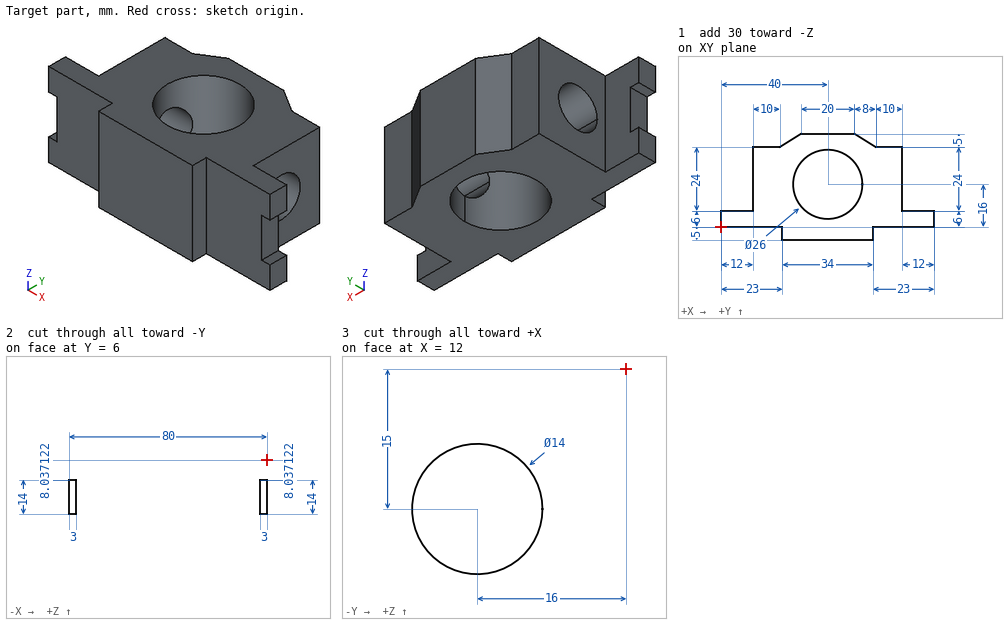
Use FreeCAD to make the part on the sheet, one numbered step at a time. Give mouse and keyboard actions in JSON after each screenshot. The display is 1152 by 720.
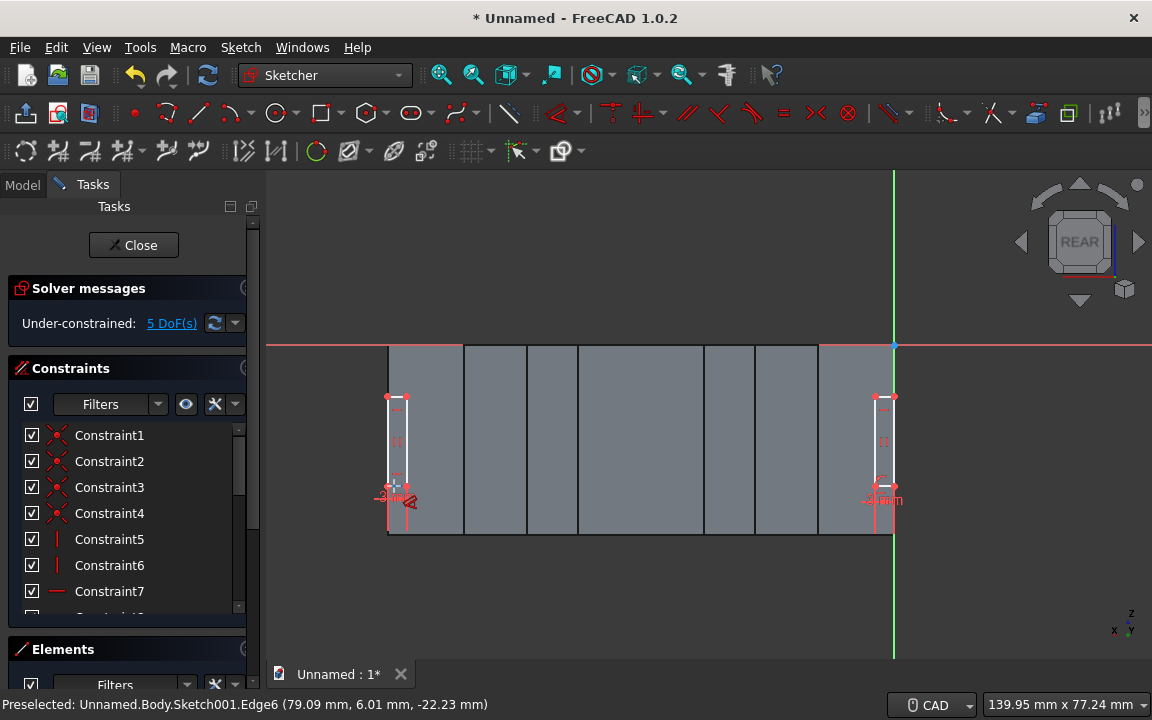
{"action": "left_click", "coordinate": [875, 424]}
{"action": "left_click", "coordinate": [909, 442]}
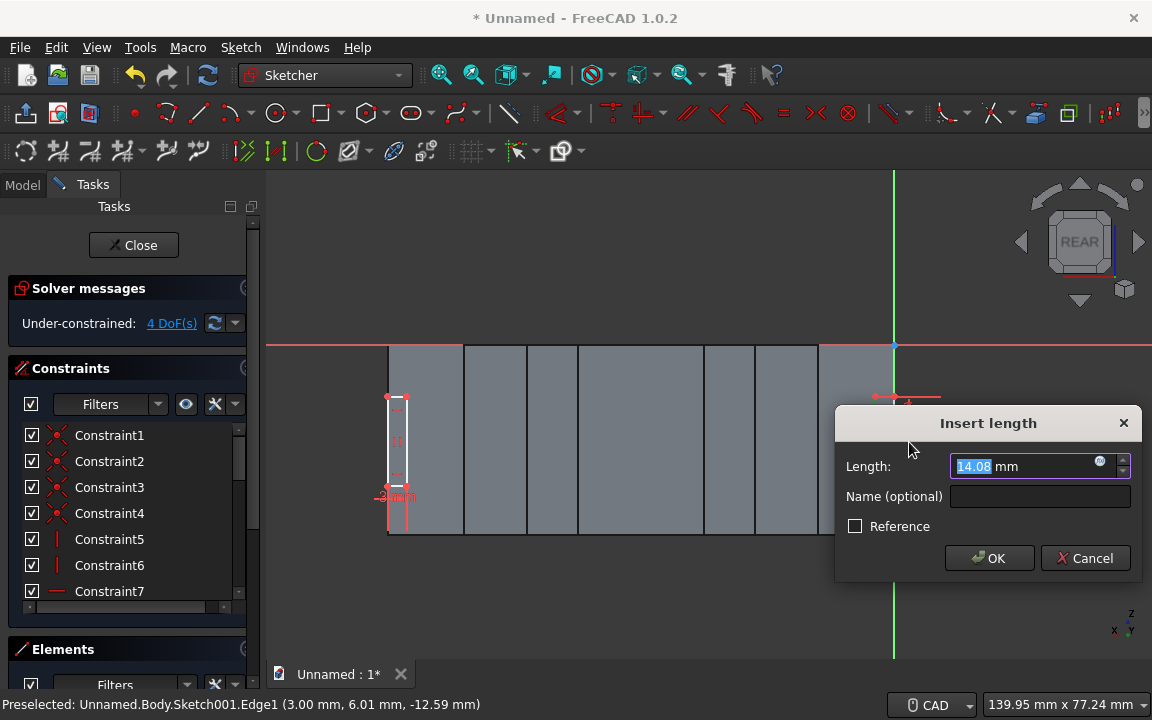
{"action": "type", "text": "14"}
{"action": "key", "text": "Return"}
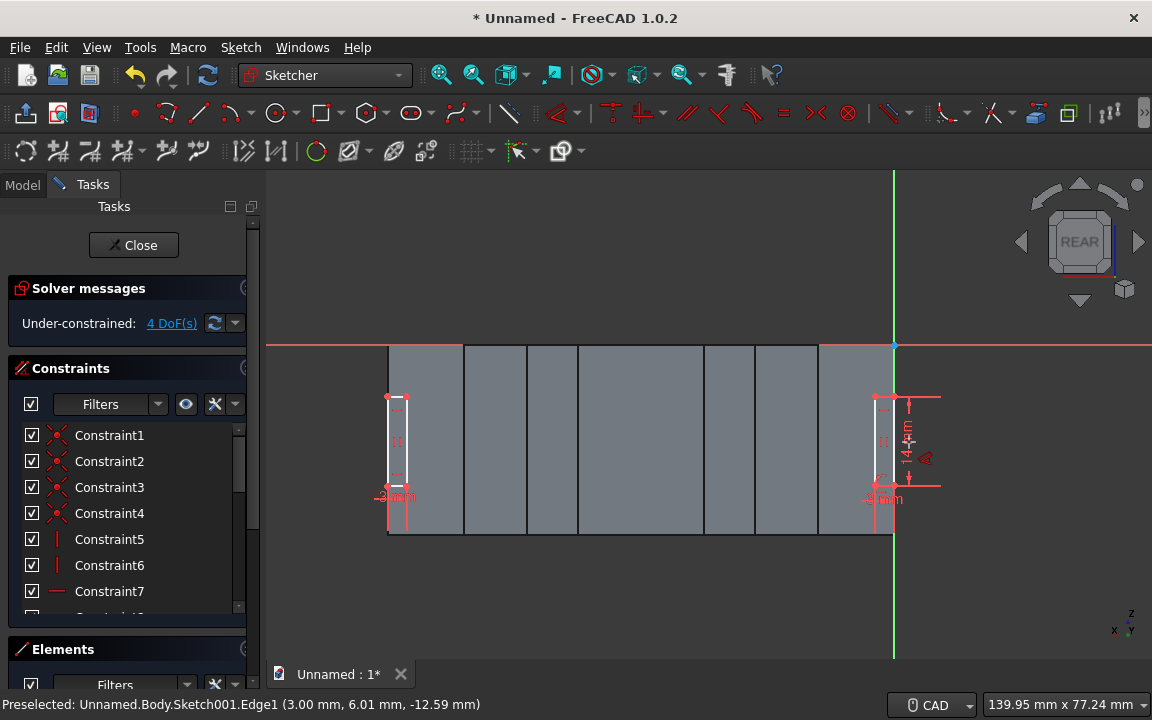
{"action": "left_click", "coordinate": [388, 424]}
{"action": "left_click", "coordinate": [354, 442]}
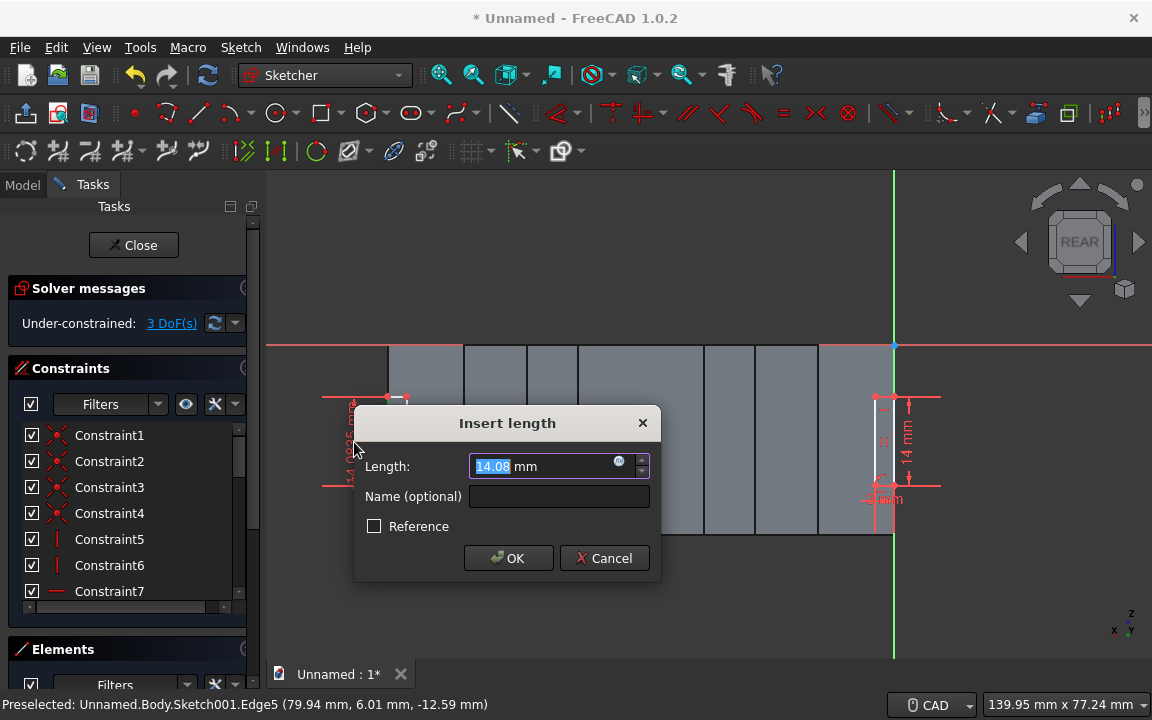
{"action": "type", "text": "14"}
{"action": "key", "text": "Return"}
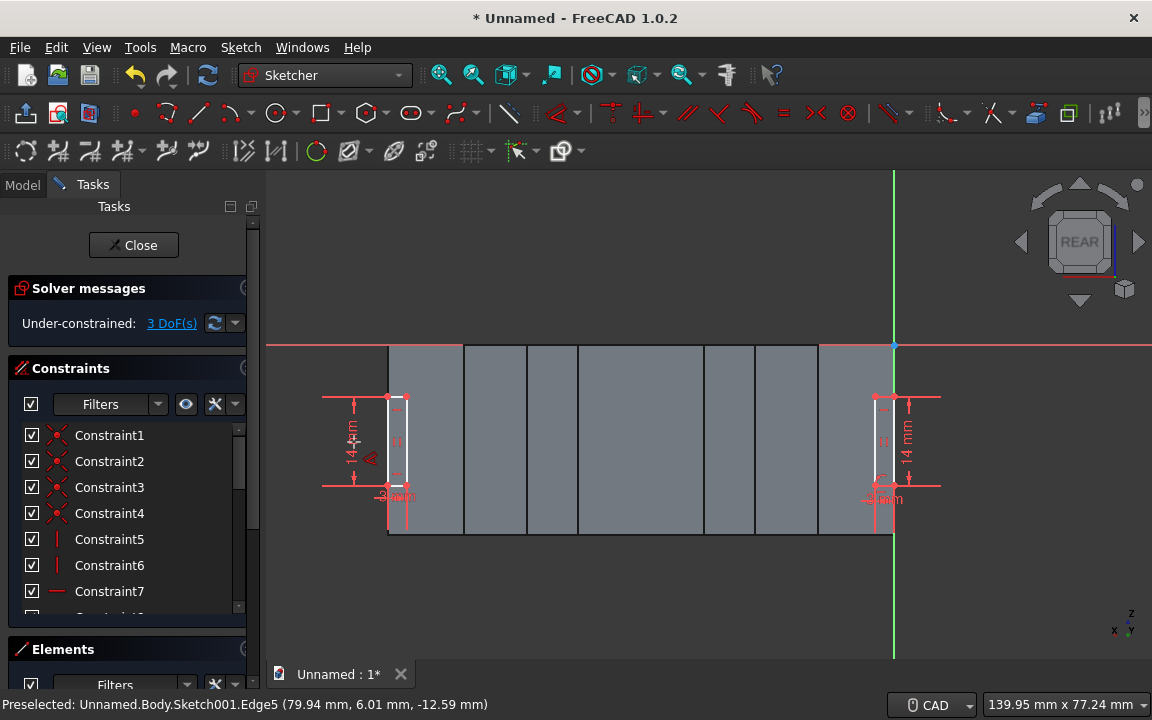
{"action": "left_click", "coordinate": [388, 397]}
{"action": "left_click", "coordinate": [641, 311]}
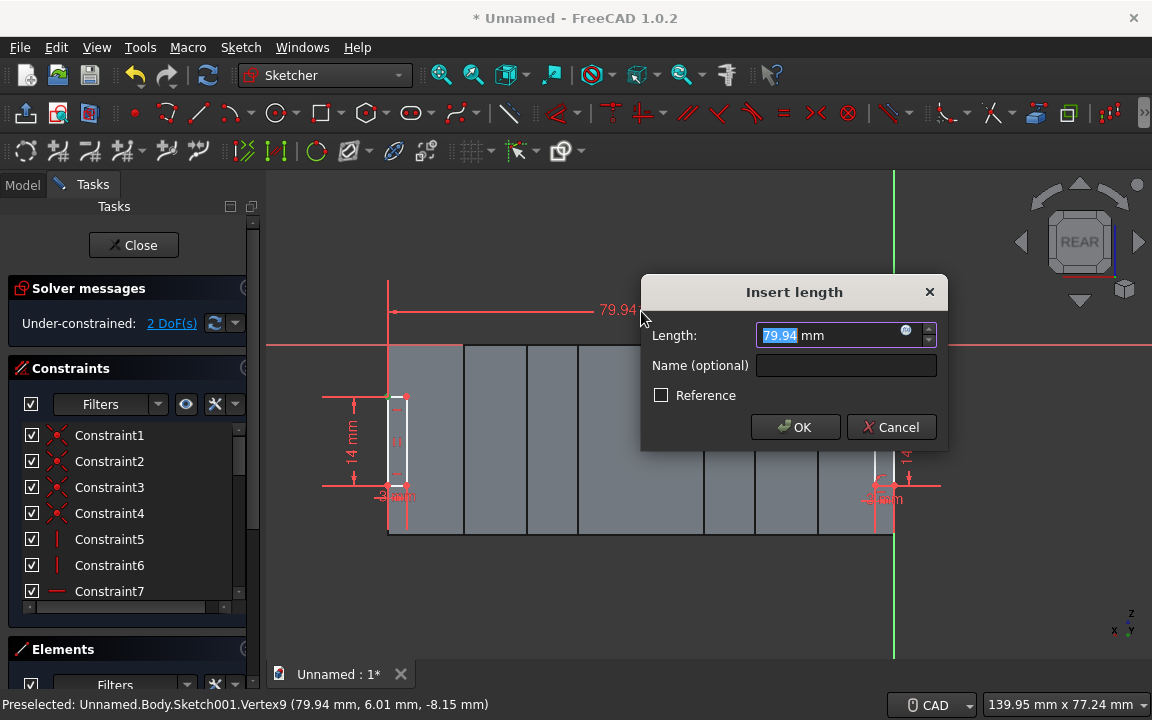
{"action": "type", "text": "80"}
{"action": "key", "text": "Return"}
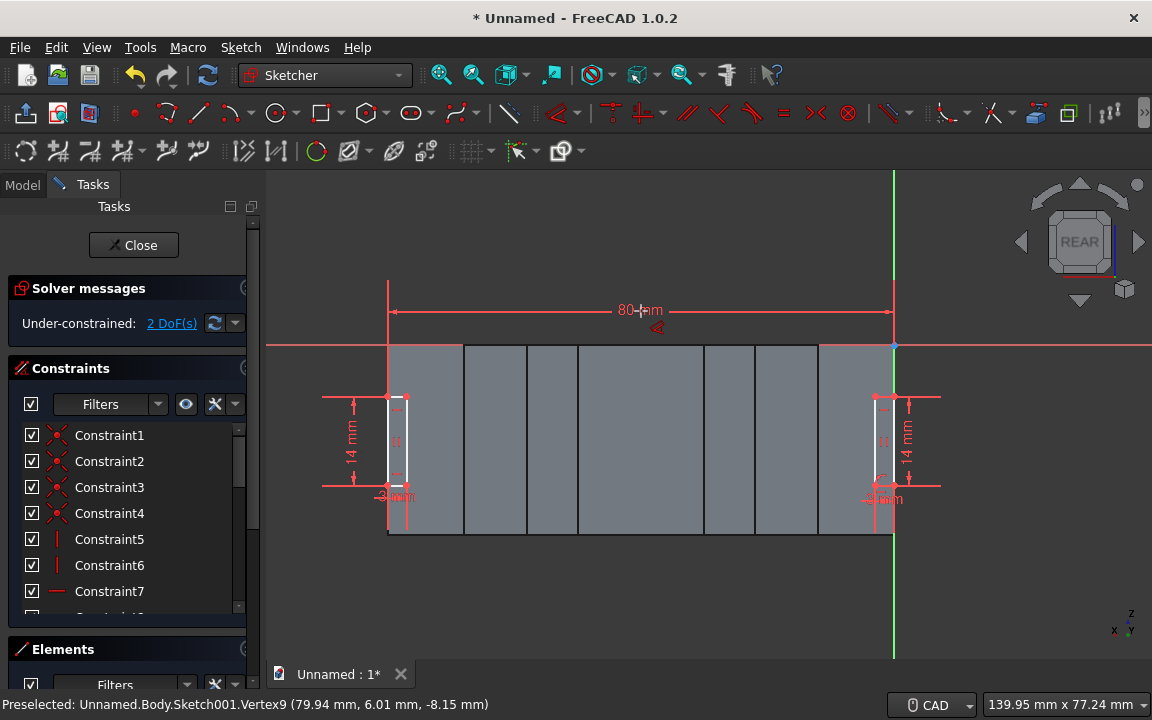
{"action": "left_click", "coordinate": [875, 397]}
{"action": "left_click", "coordinate": [928, 371]}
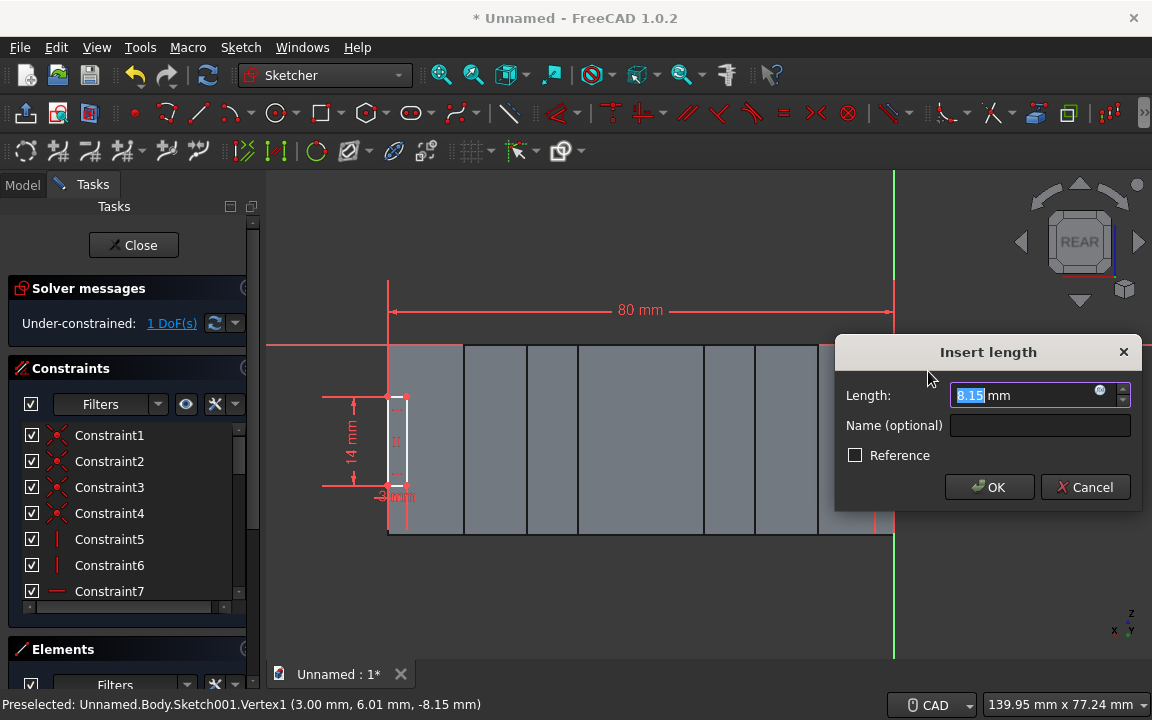
{"action": "type", "text": "8.037122"}
{"action": "key", "text": "Return"}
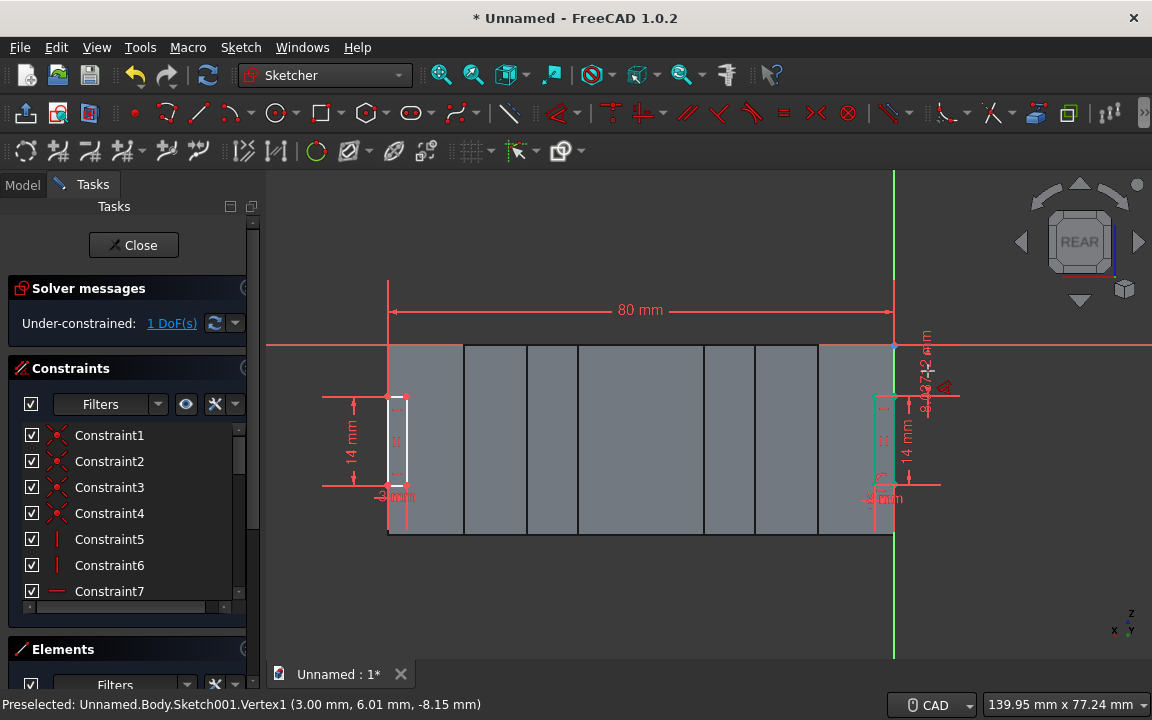
{"action": "left_click", "coordinate": [388, 397]}
{"action": "left_click", "coordinate": [354, 371]}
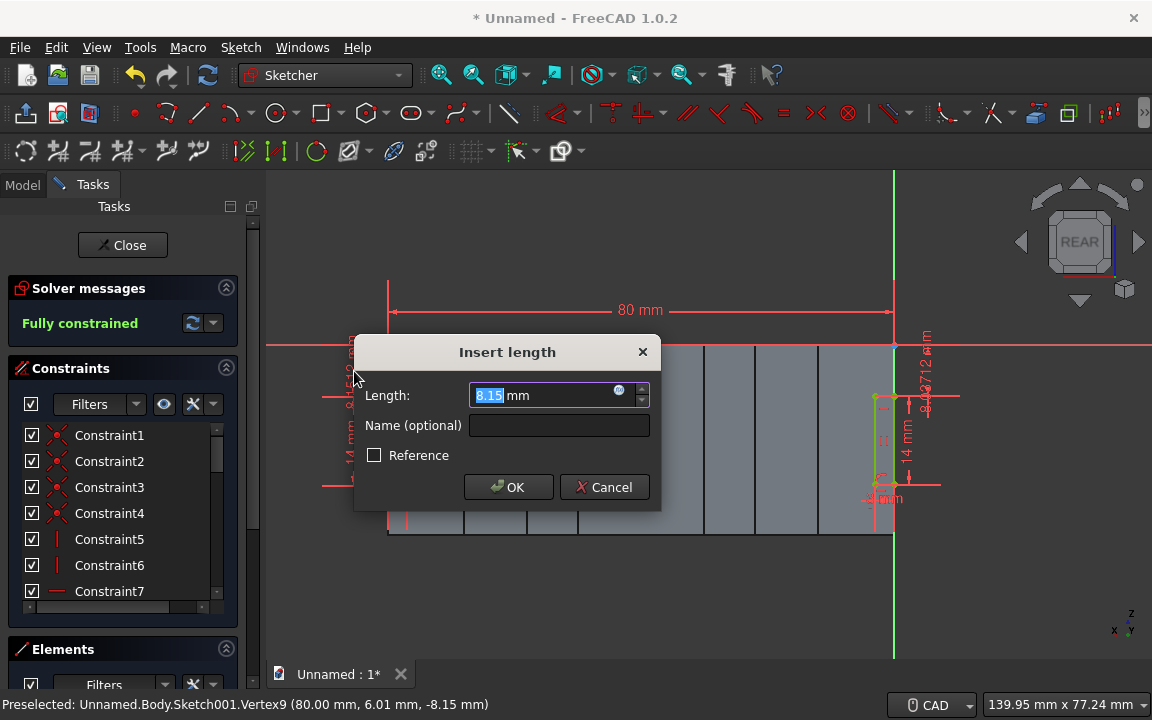
{"action": "type", "text": "8.037122"}
{"action": "key", "text": "Return"}
{"action": "key", "text": "Escape"}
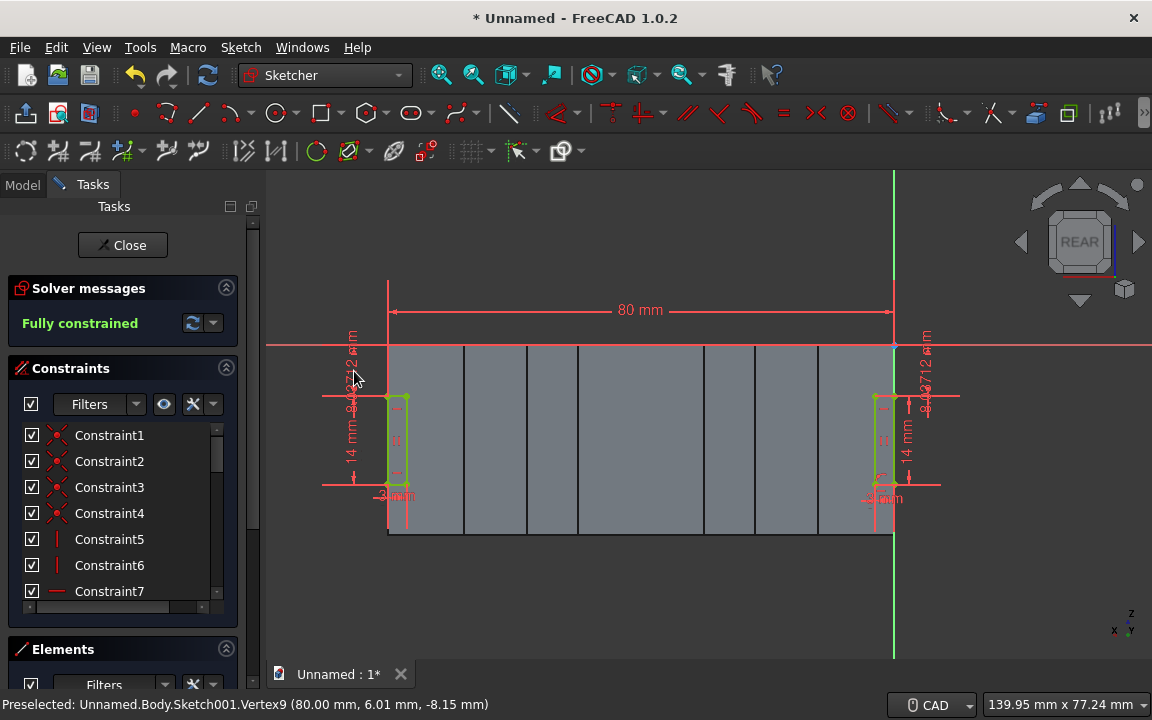
{"action": "left_click", "coordinate": [123, 245]}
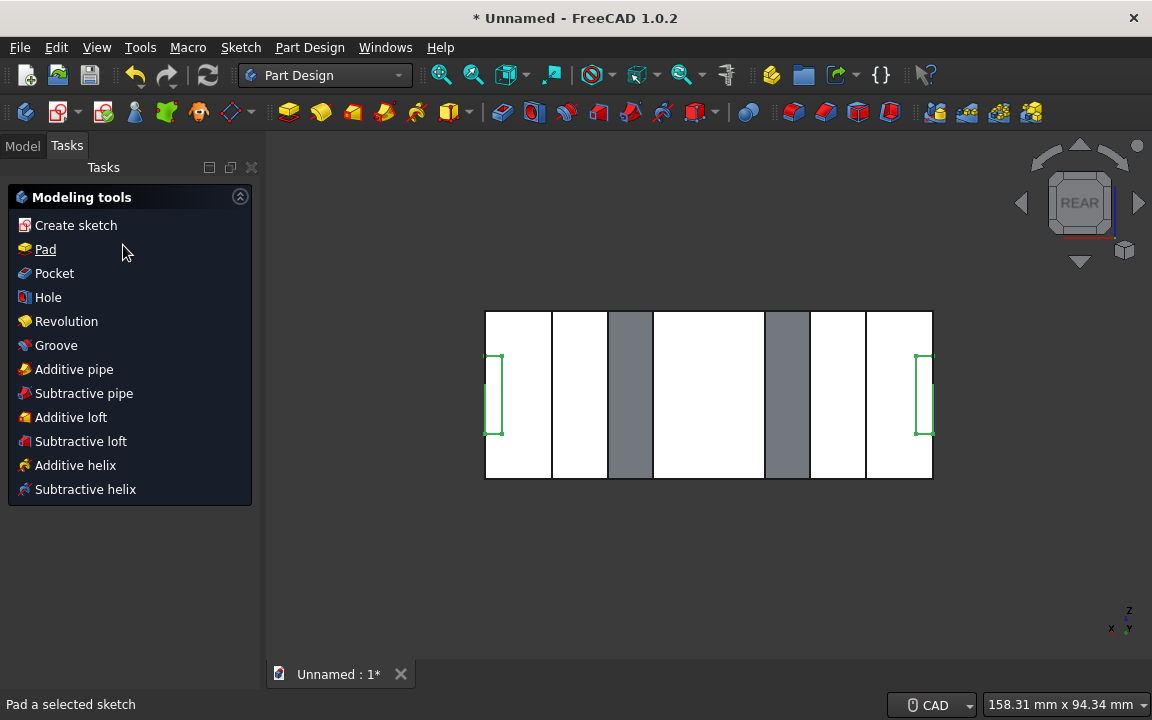
{"action": "left_click", "coordinate": [504, 112]}